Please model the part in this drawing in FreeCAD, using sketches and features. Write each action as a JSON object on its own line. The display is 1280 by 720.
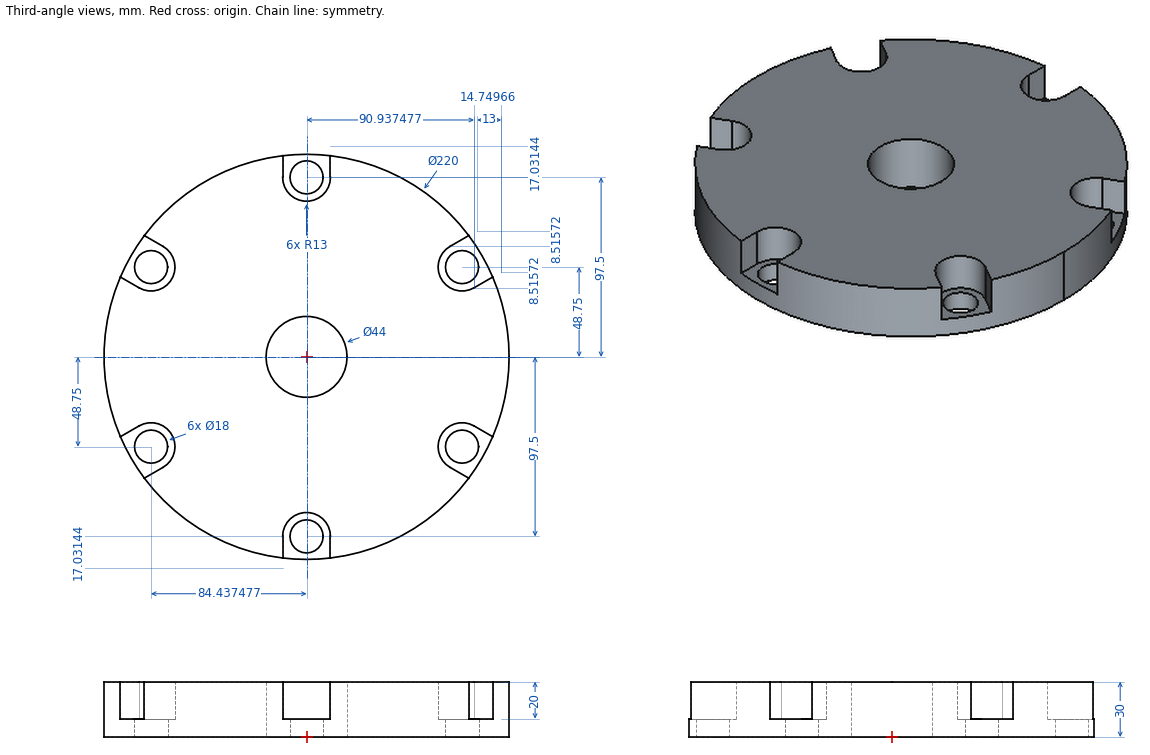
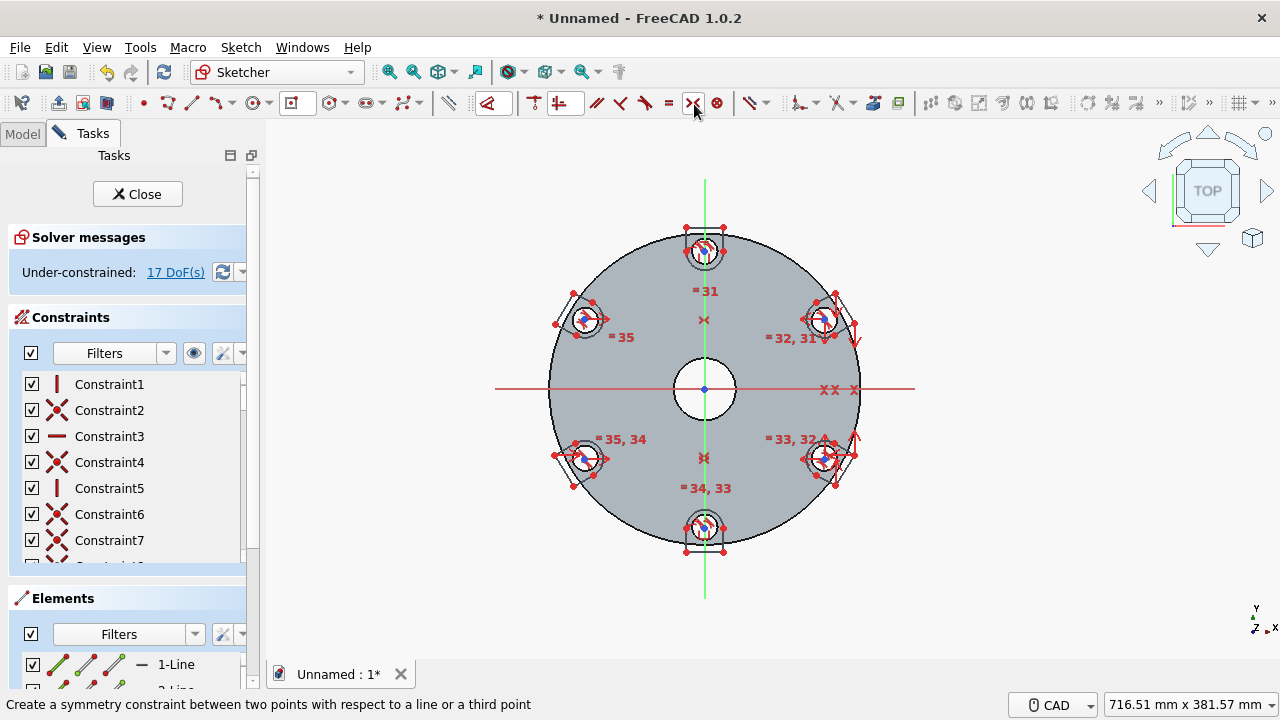
{"action": "left_click", "coordinate": [836, 485]}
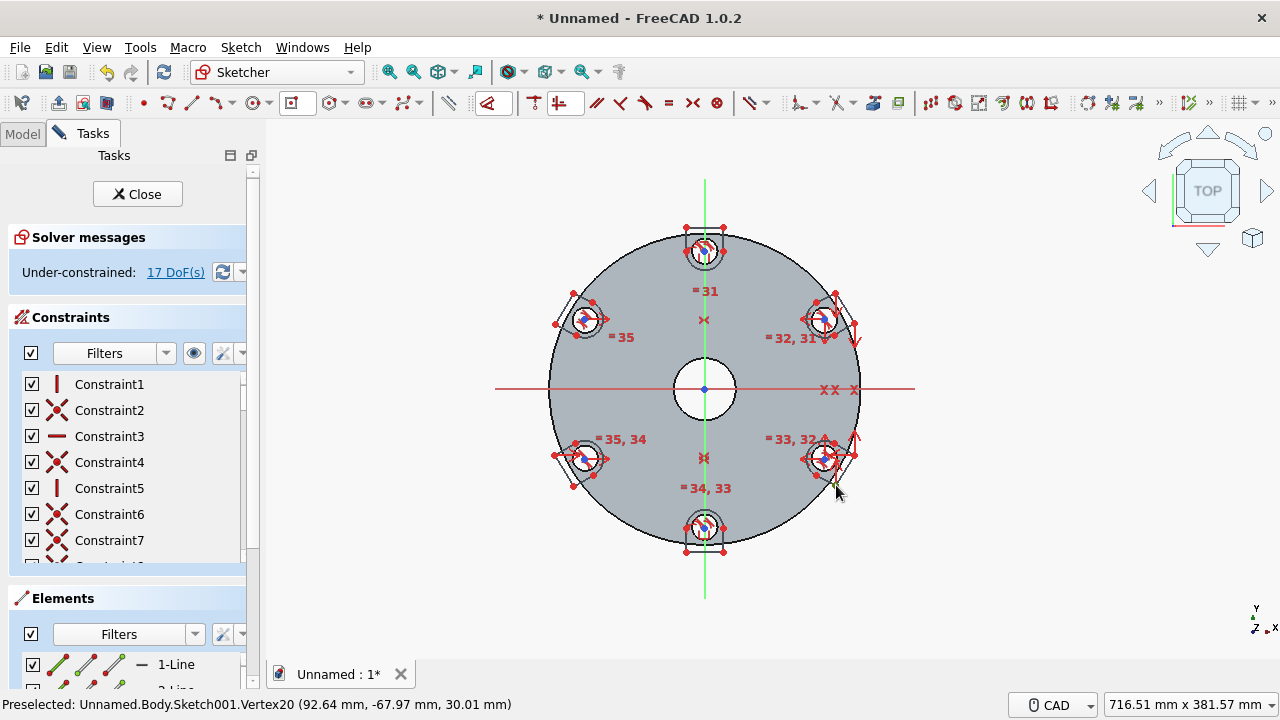
{"action": "left_click", "coordinate": [574, 487]}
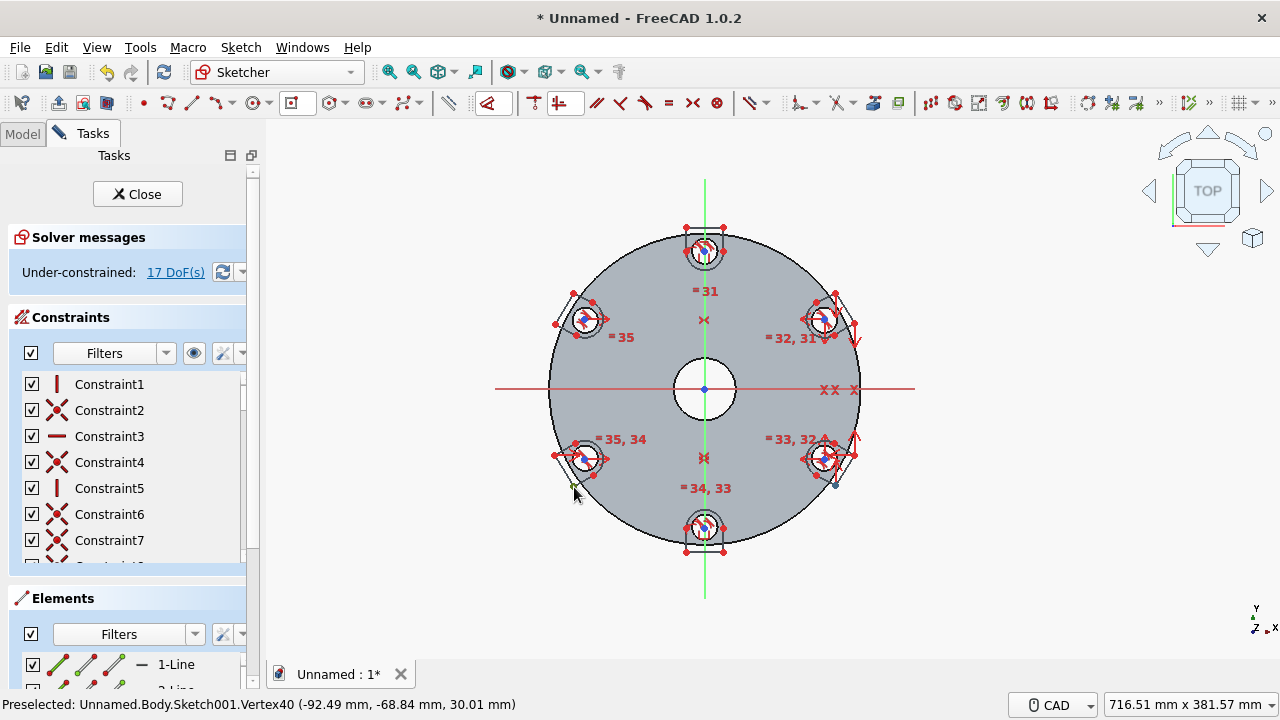
{"action": "left_click", "coordinate": [705, 596]}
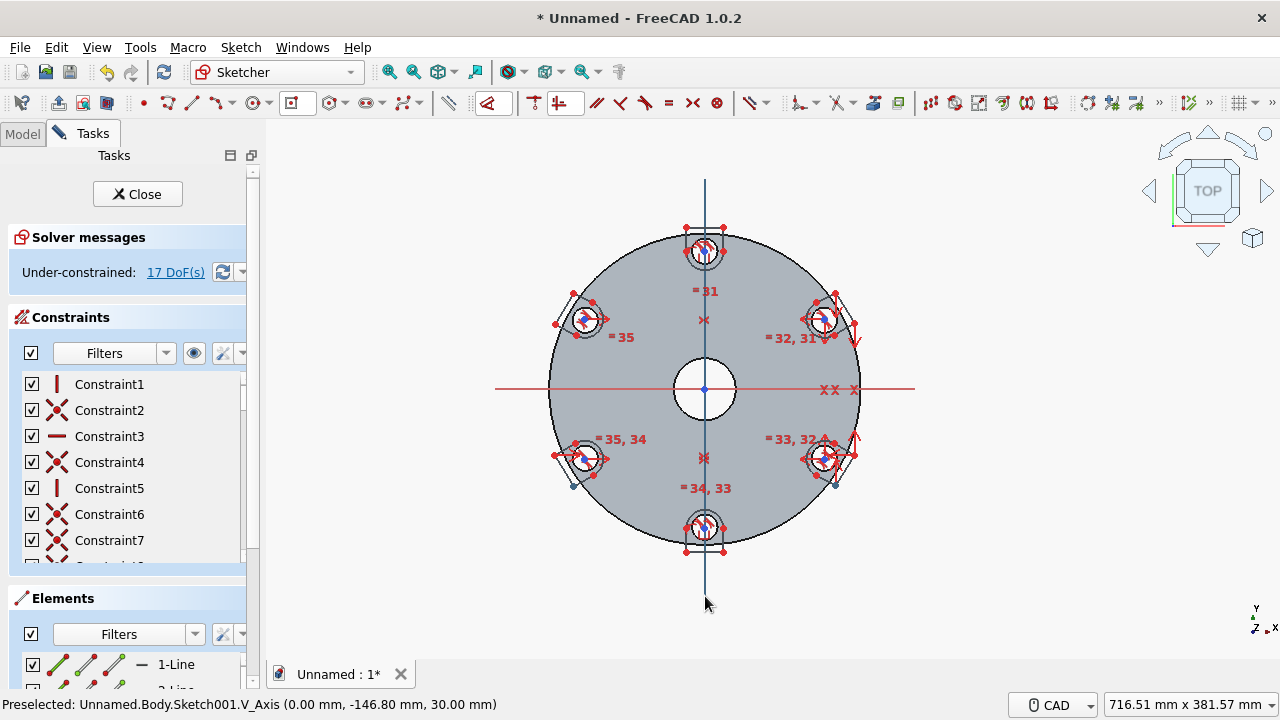
{"action": "left_click", "coordinate": [694, 104]}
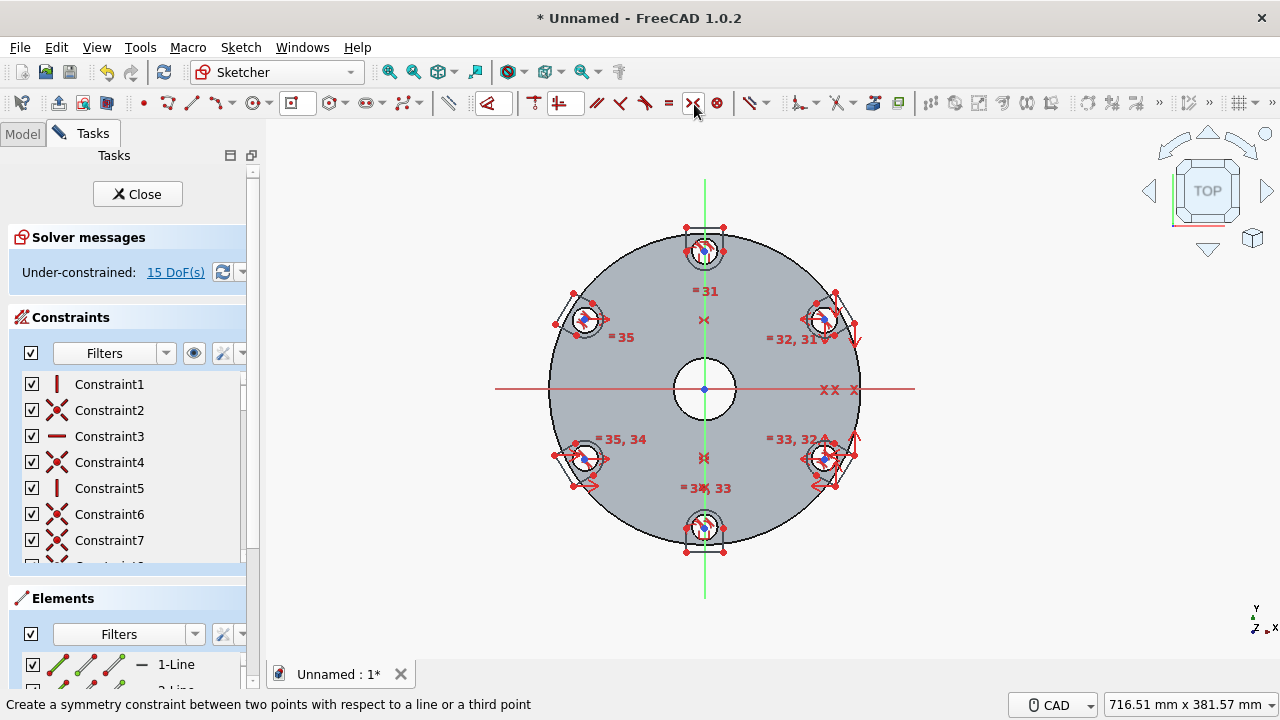
{"action": "left_click", "coordinate": [836, 292]}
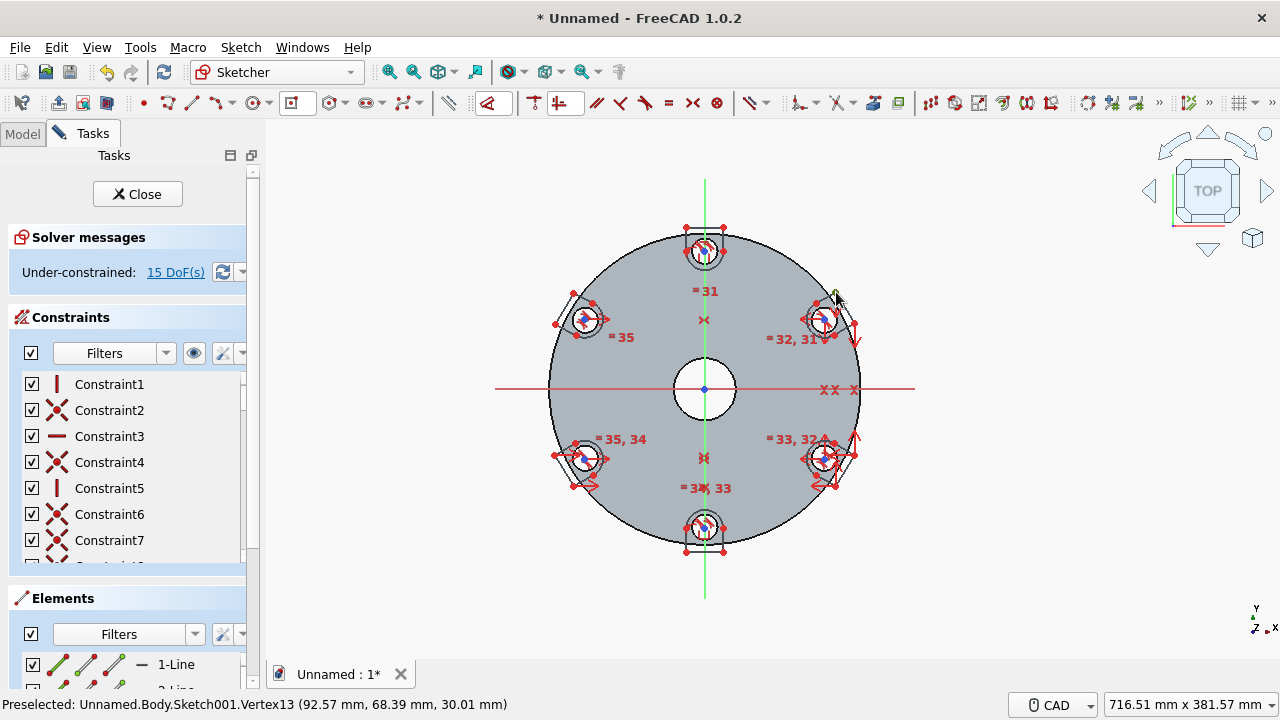
{"action": "left_click", "coordinate": [574, 293]}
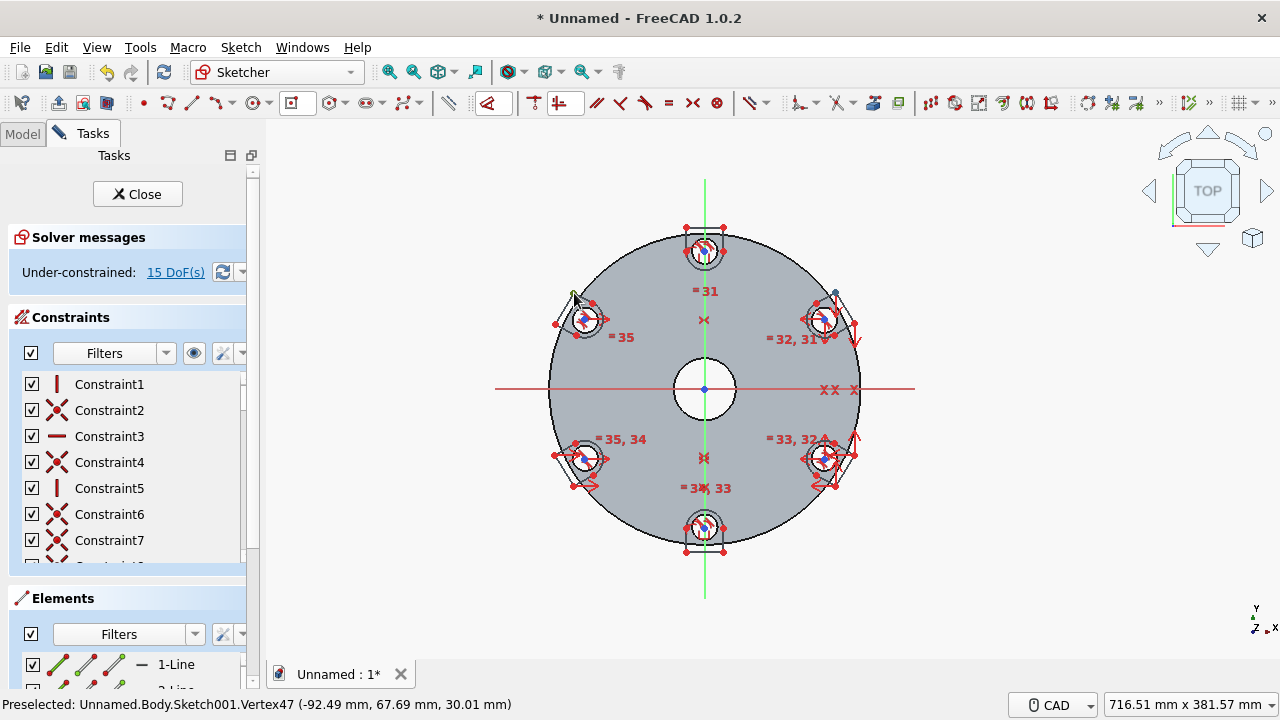
{"action": "left_click", "coordinate": [705, 596]}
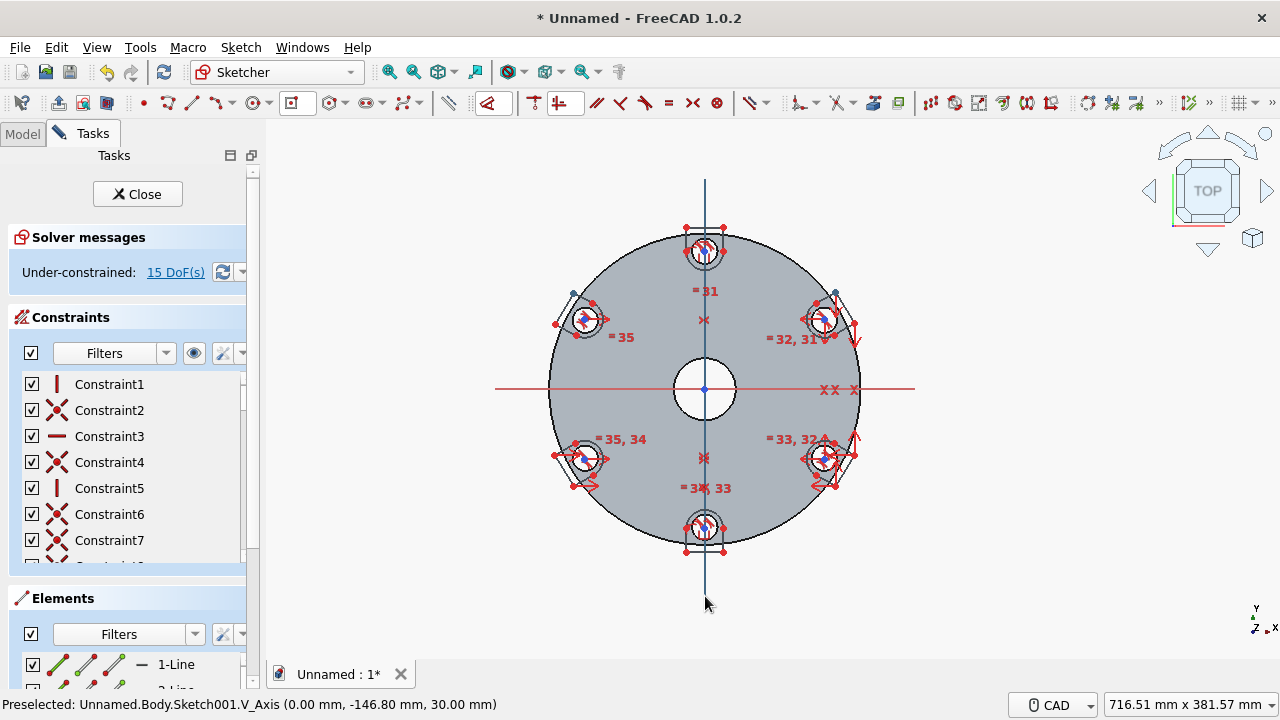
{"action": "left_click", "coordinate": [694, 104]}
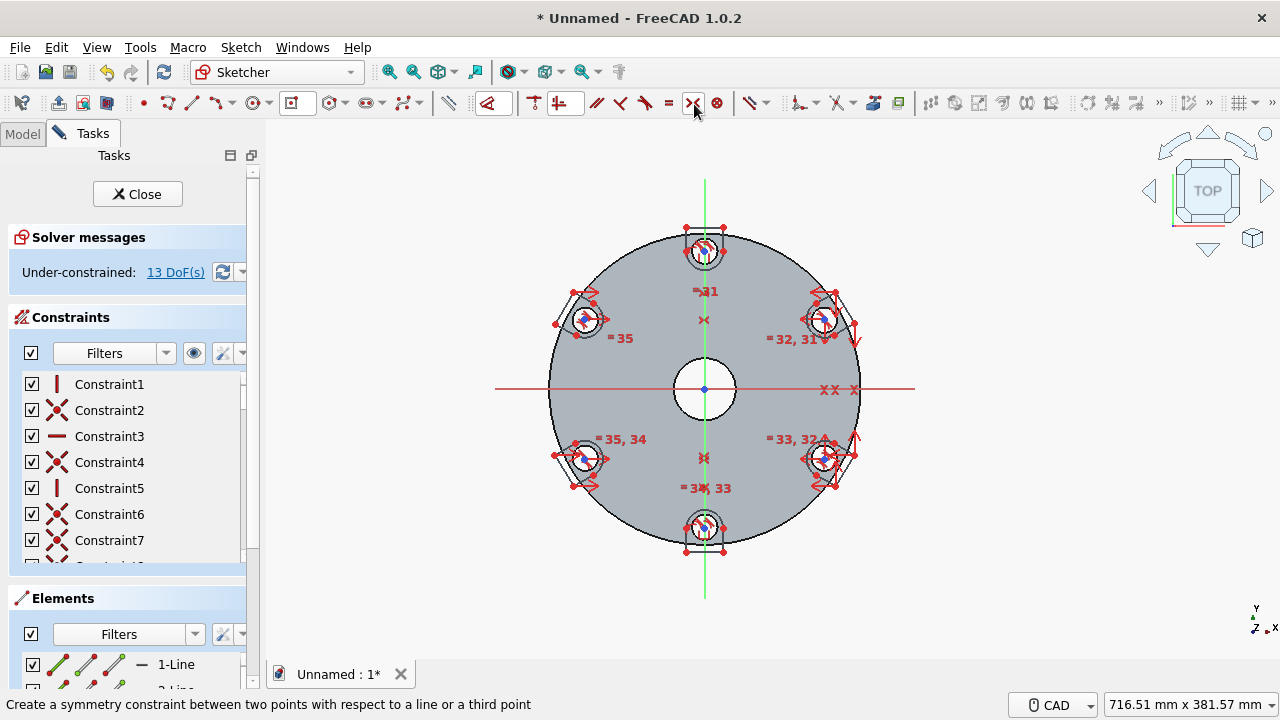
{"action": "left_click", "coordinate": [855, 323]}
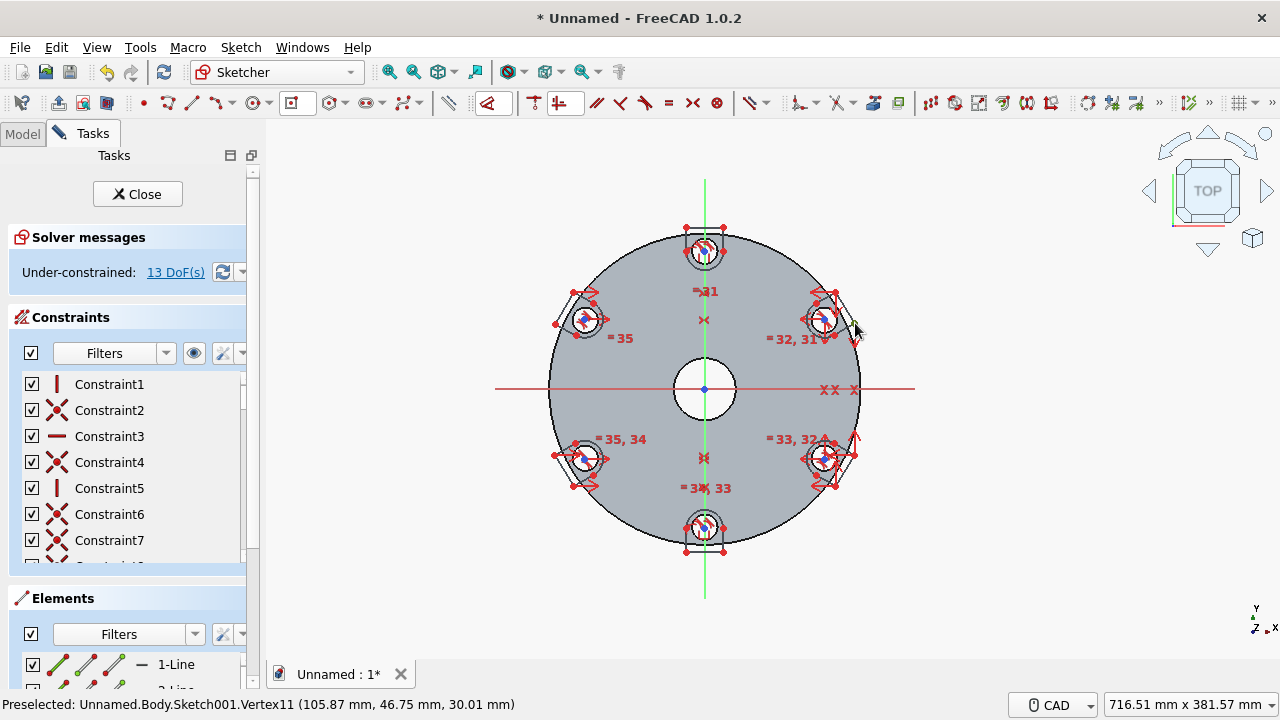
{"action": "left_click", "coordinate": [555, 325]}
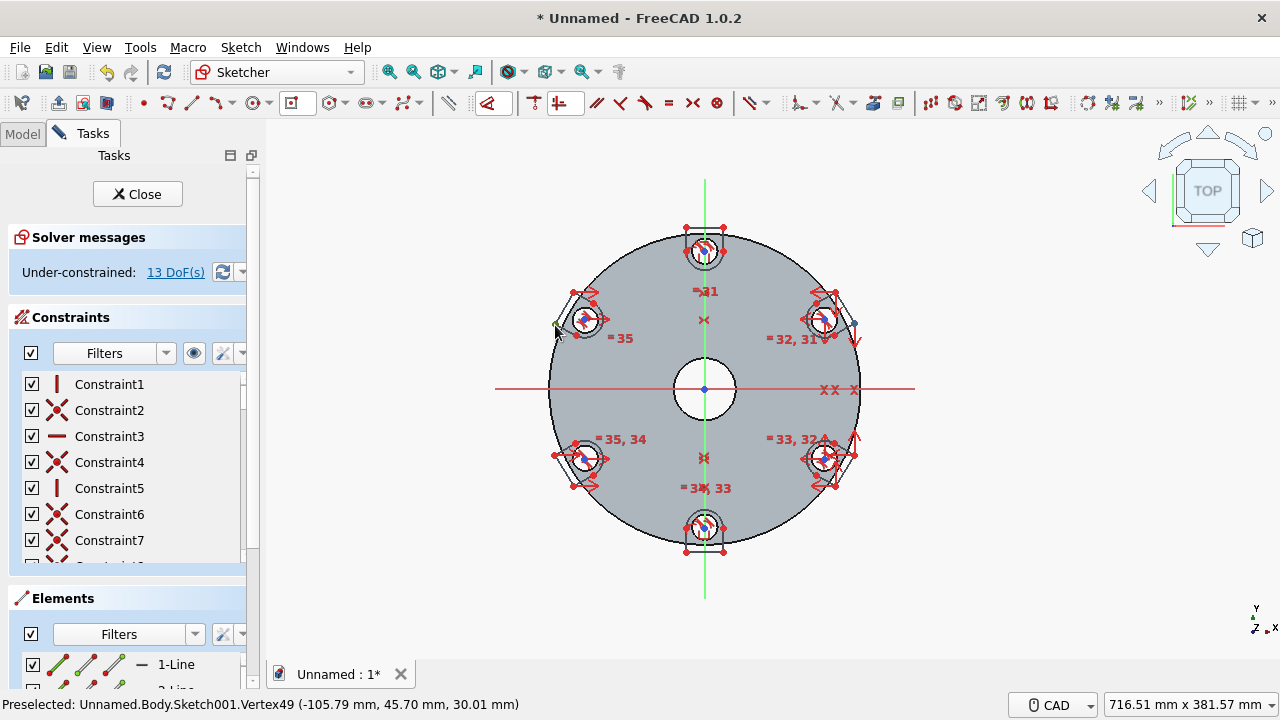
{"action": "left_click", "coordinate": [705, 596]}